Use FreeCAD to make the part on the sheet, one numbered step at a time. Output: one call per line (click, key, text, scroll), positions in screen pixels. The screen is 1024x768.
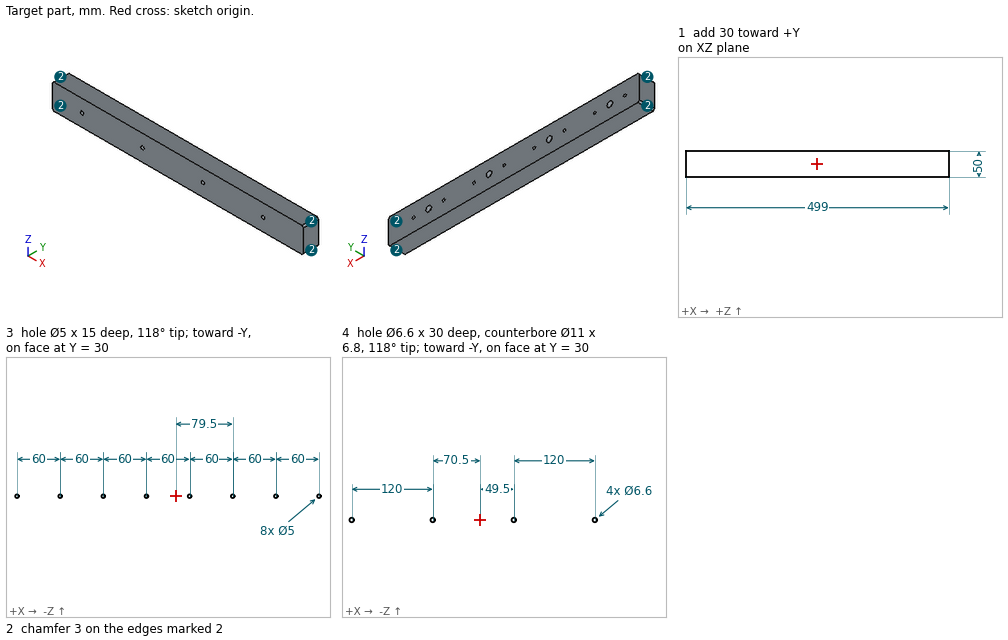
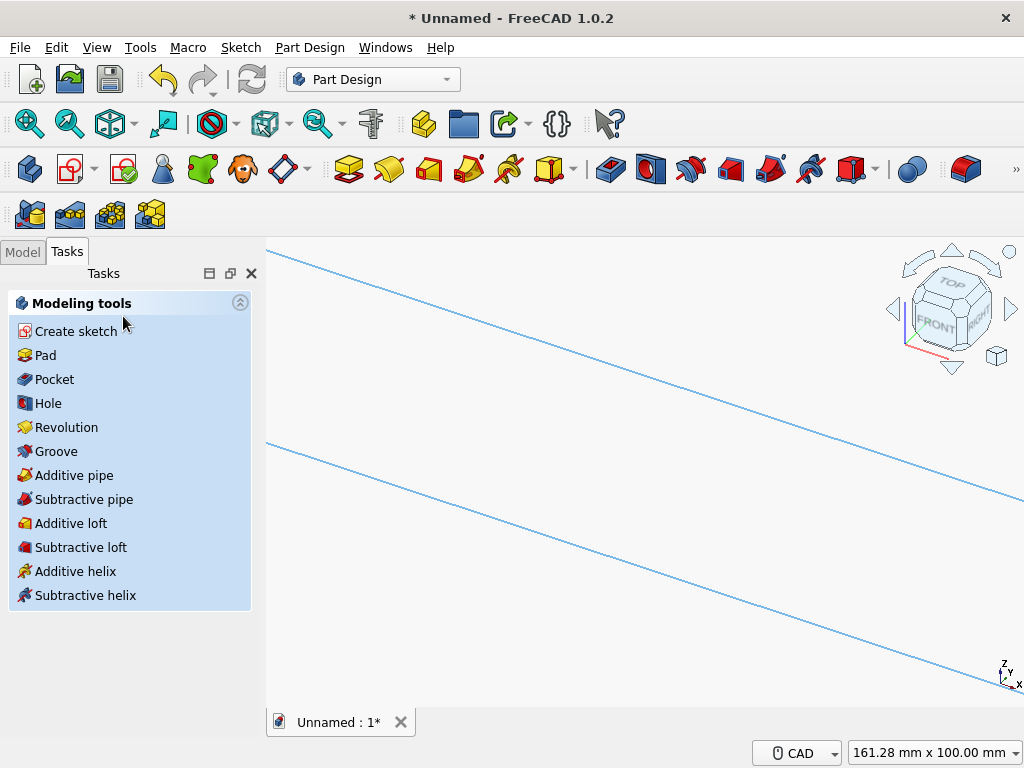
click(350, 170)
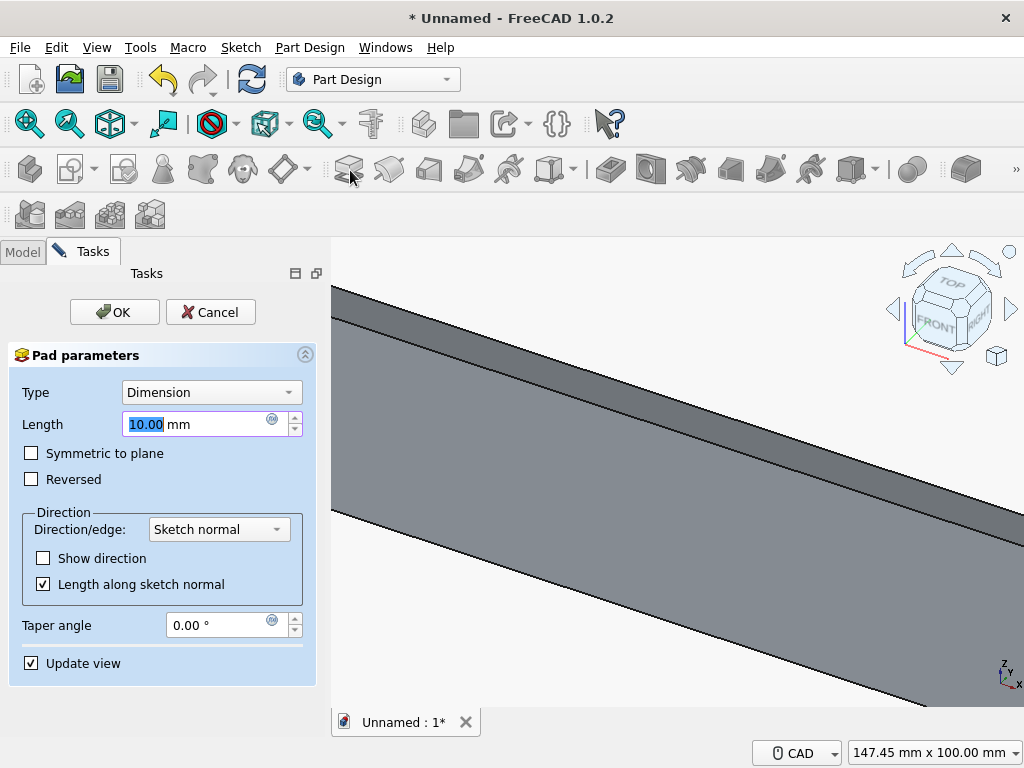
text(30)
key(Tab)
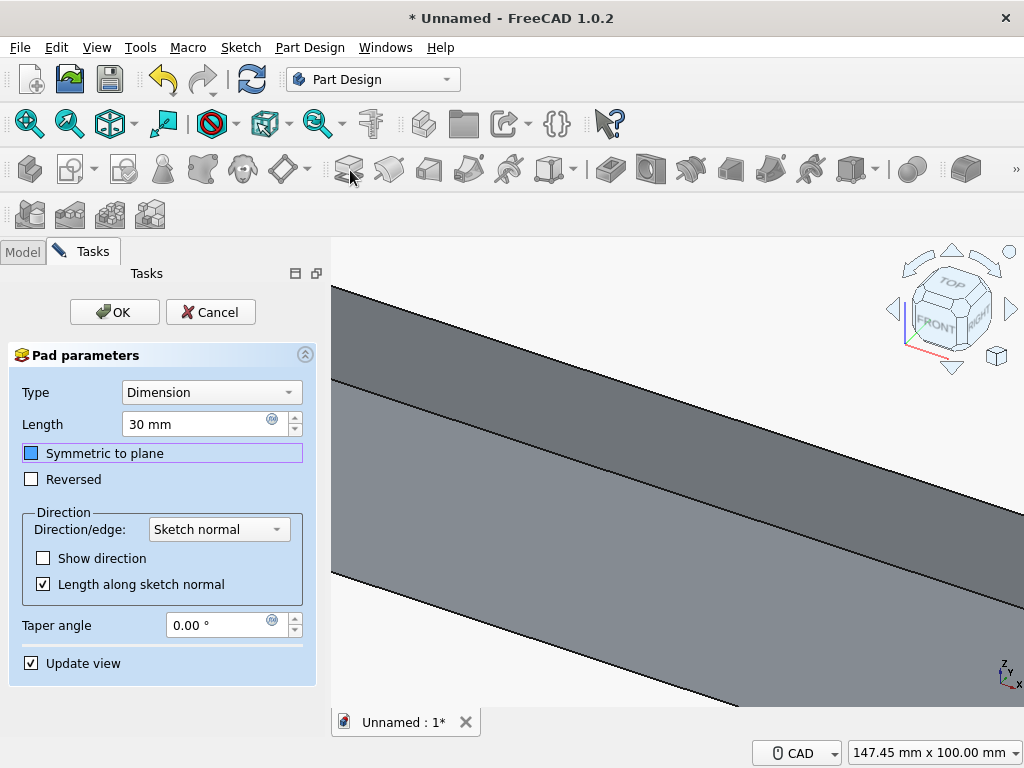
click(30, 479)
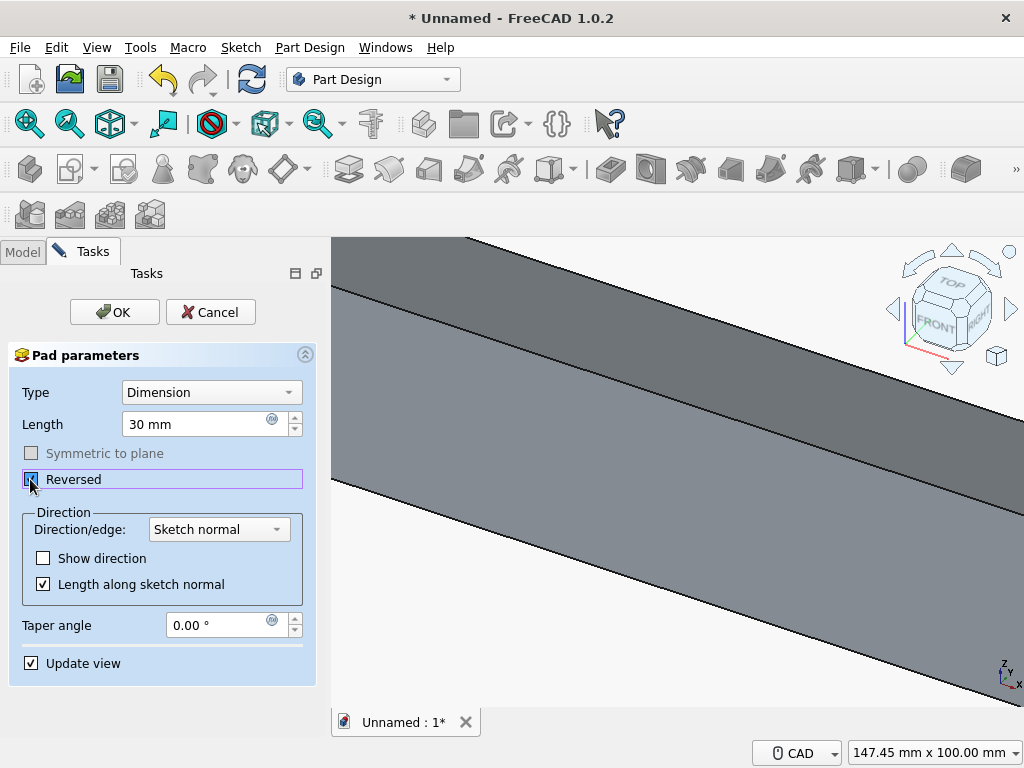
click(115, 312)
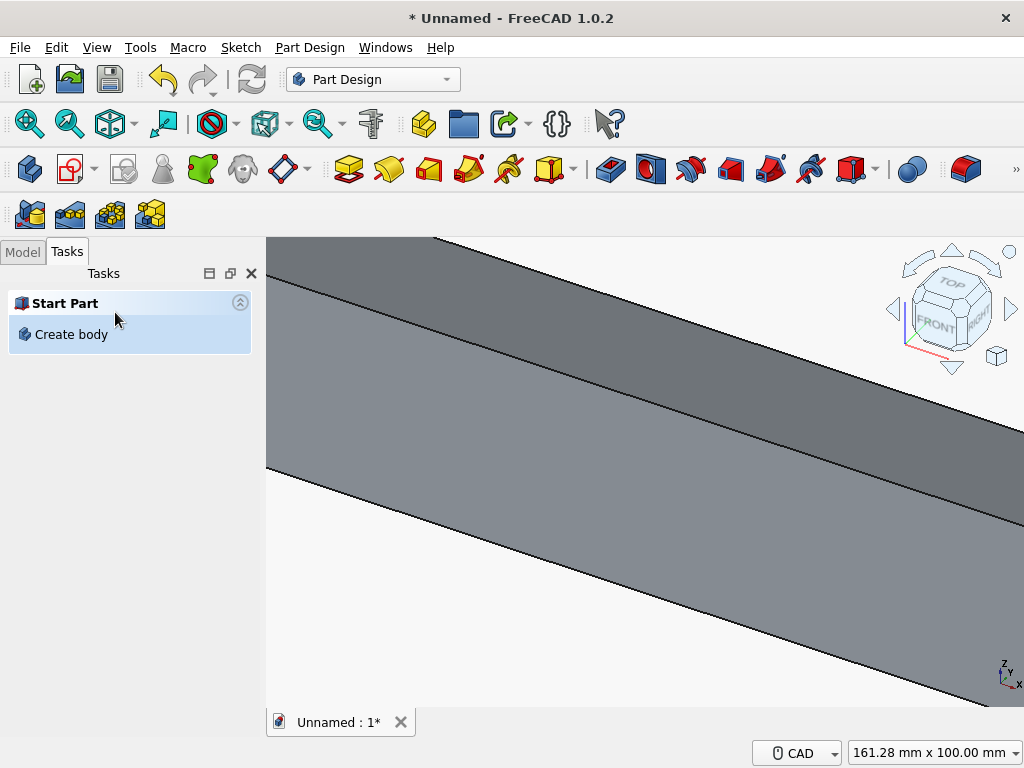
click(30, 124)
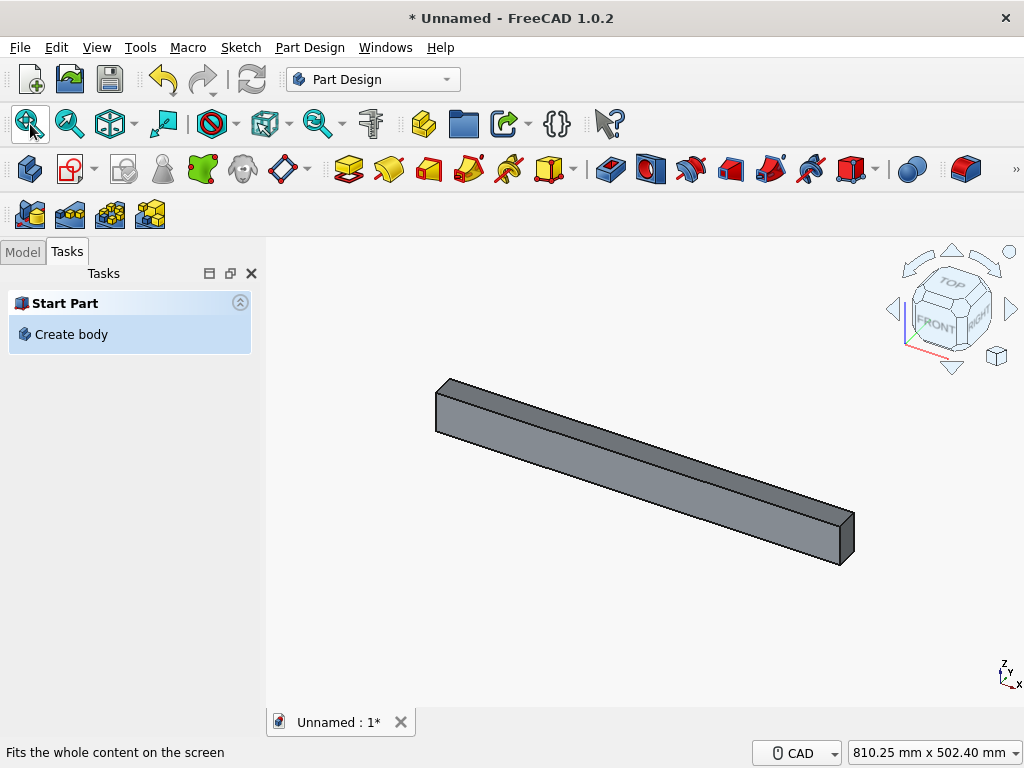
click(847, 519)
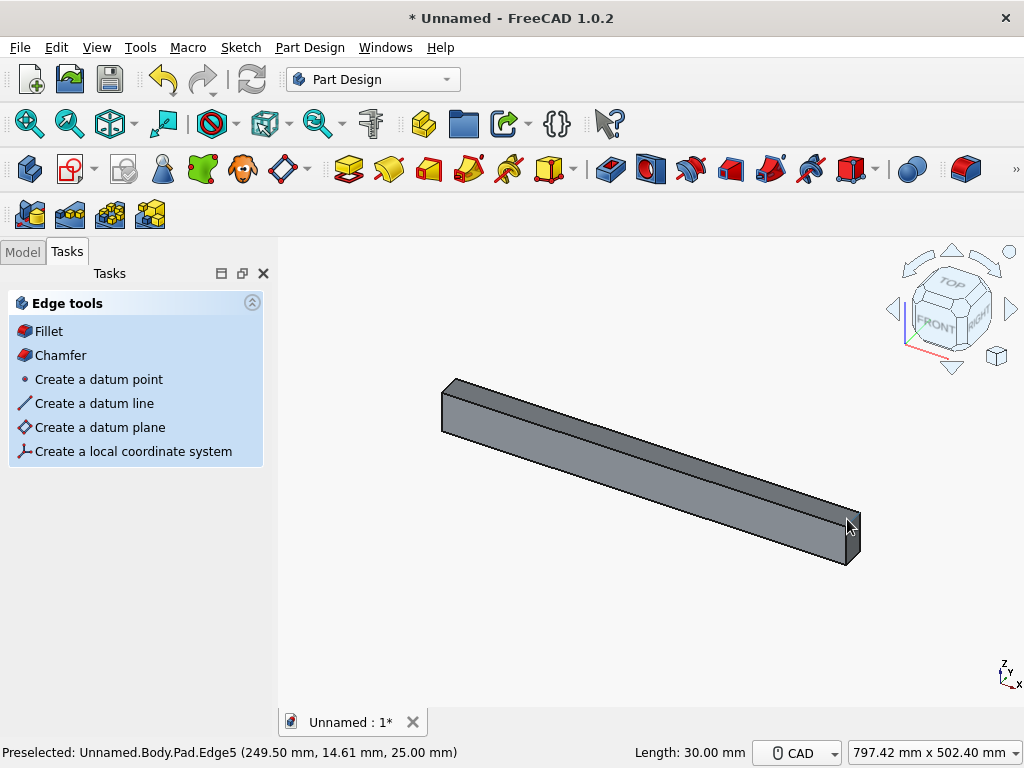
key(0)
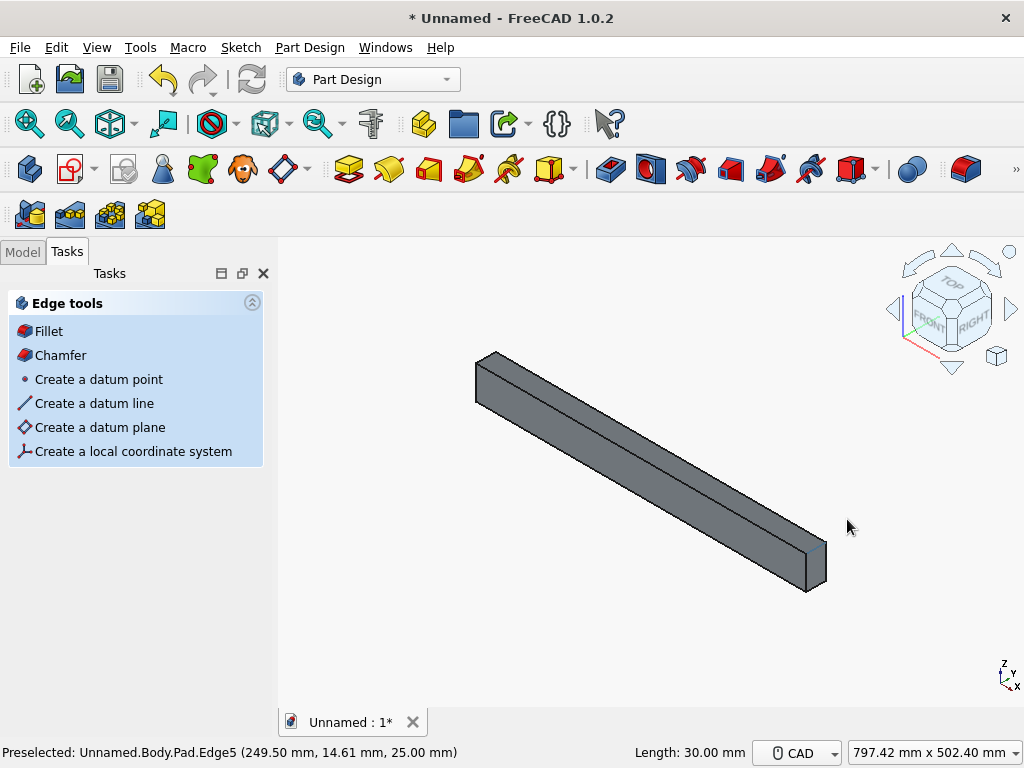
key(2)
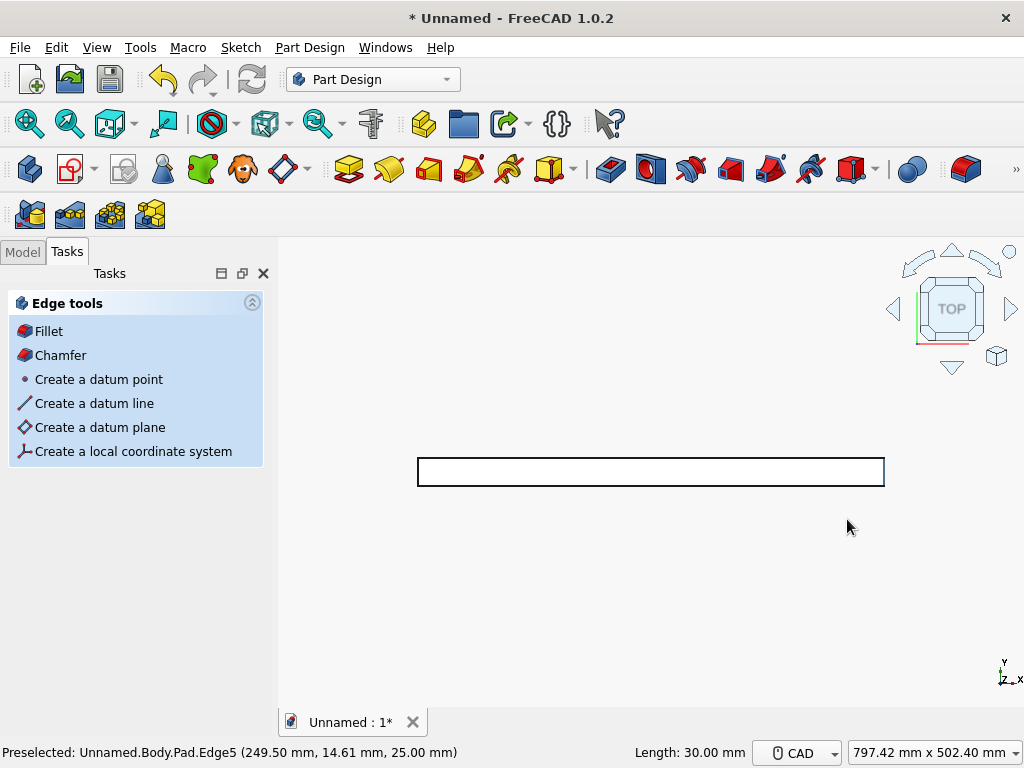
click(418, 471, ctrl)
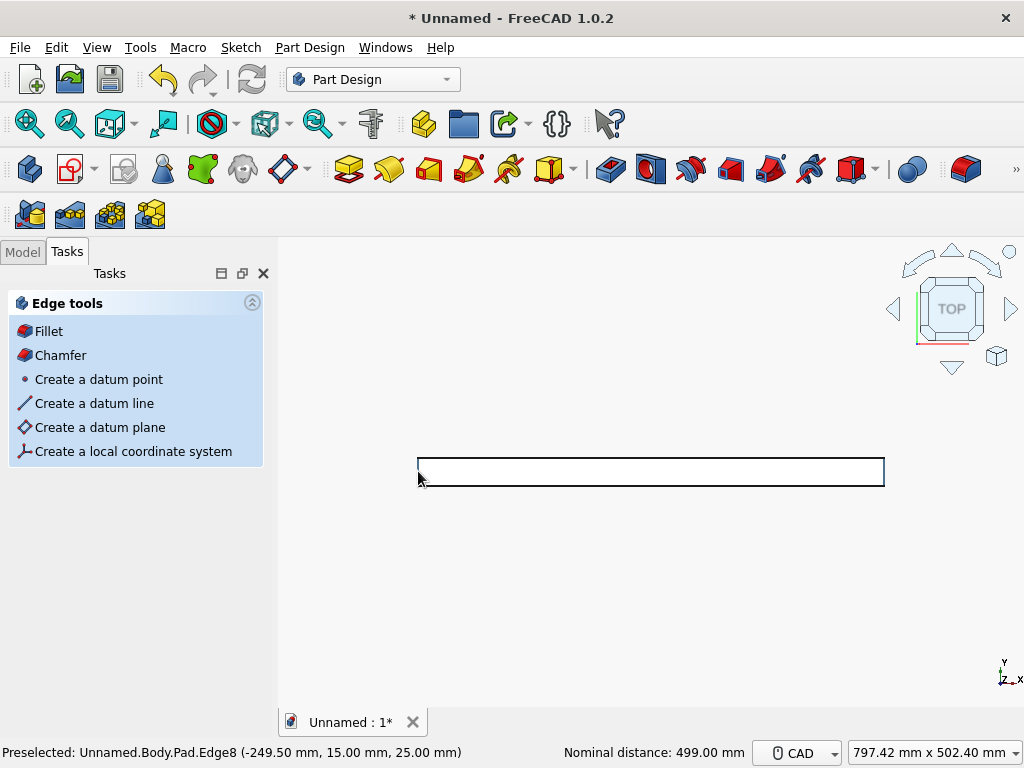
key(1)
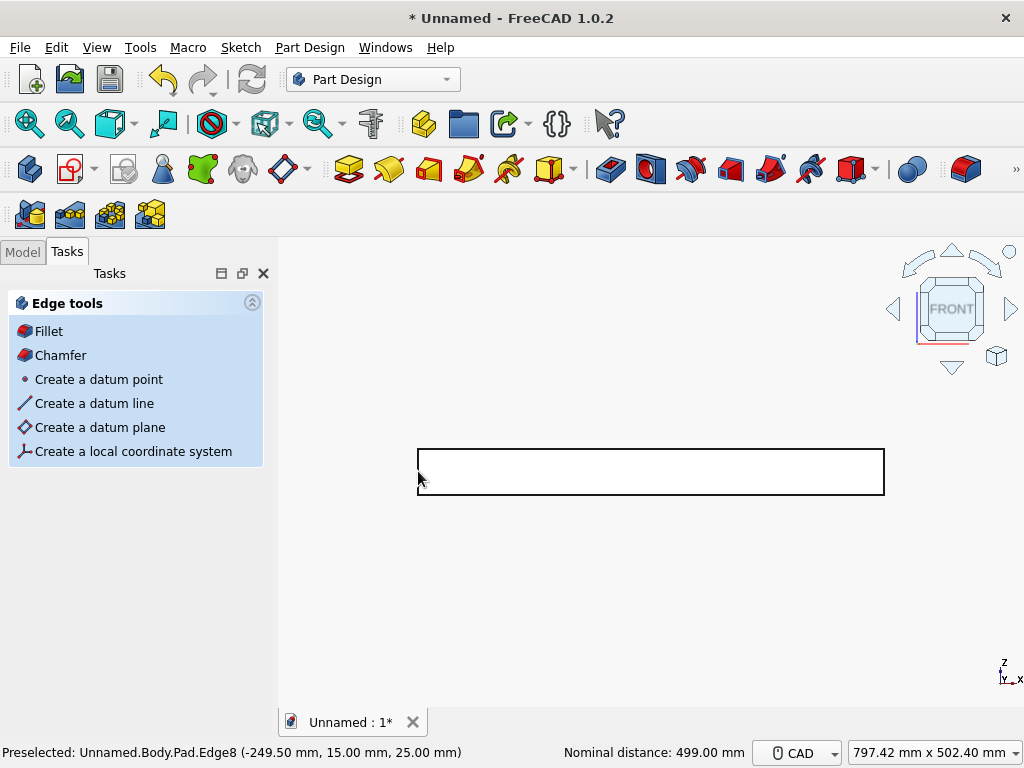
key(3)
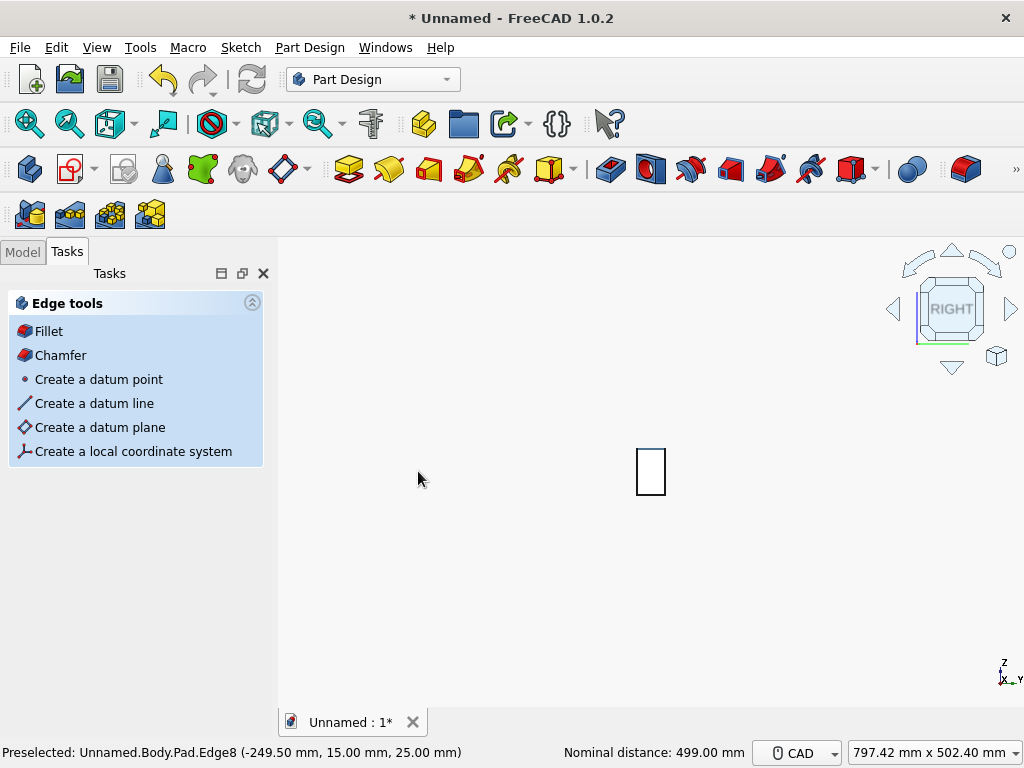
key(v)
key(f)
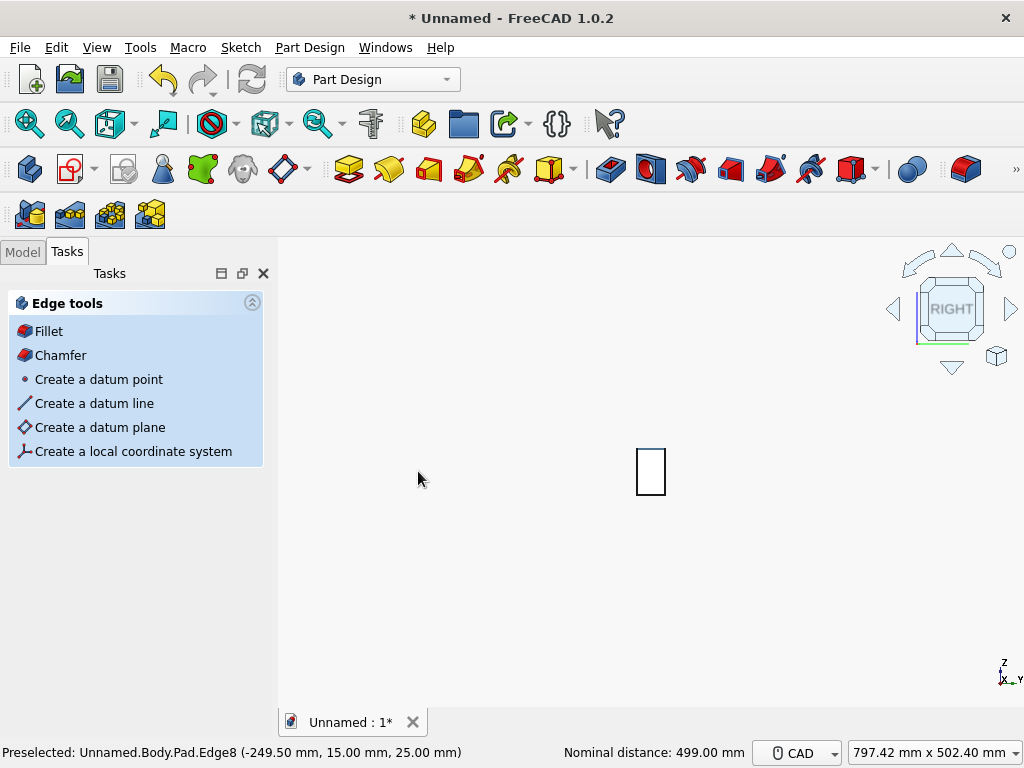
click(651, 494, ctrl)